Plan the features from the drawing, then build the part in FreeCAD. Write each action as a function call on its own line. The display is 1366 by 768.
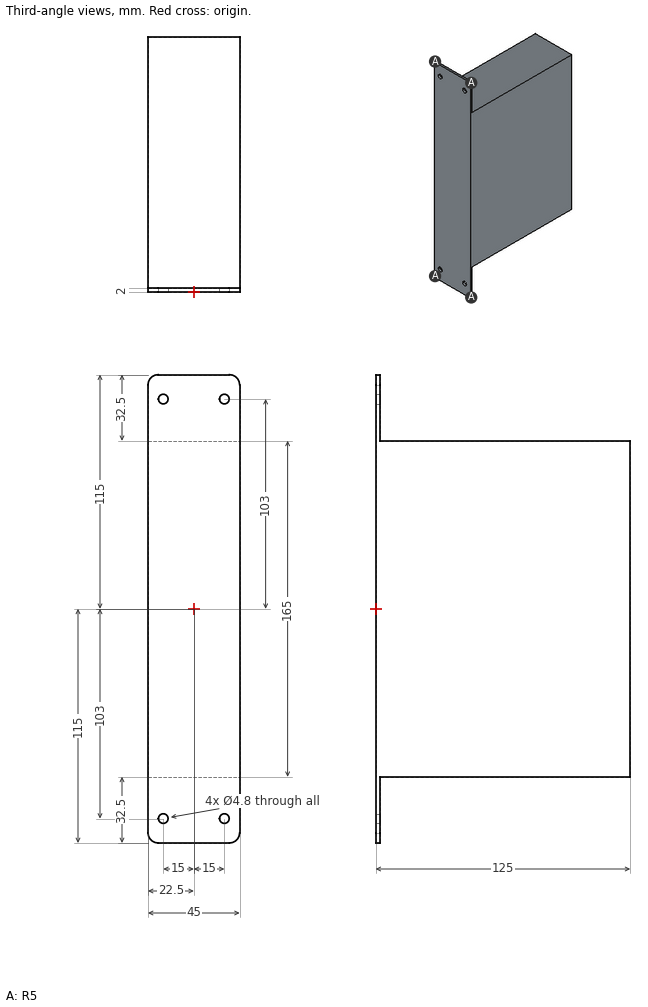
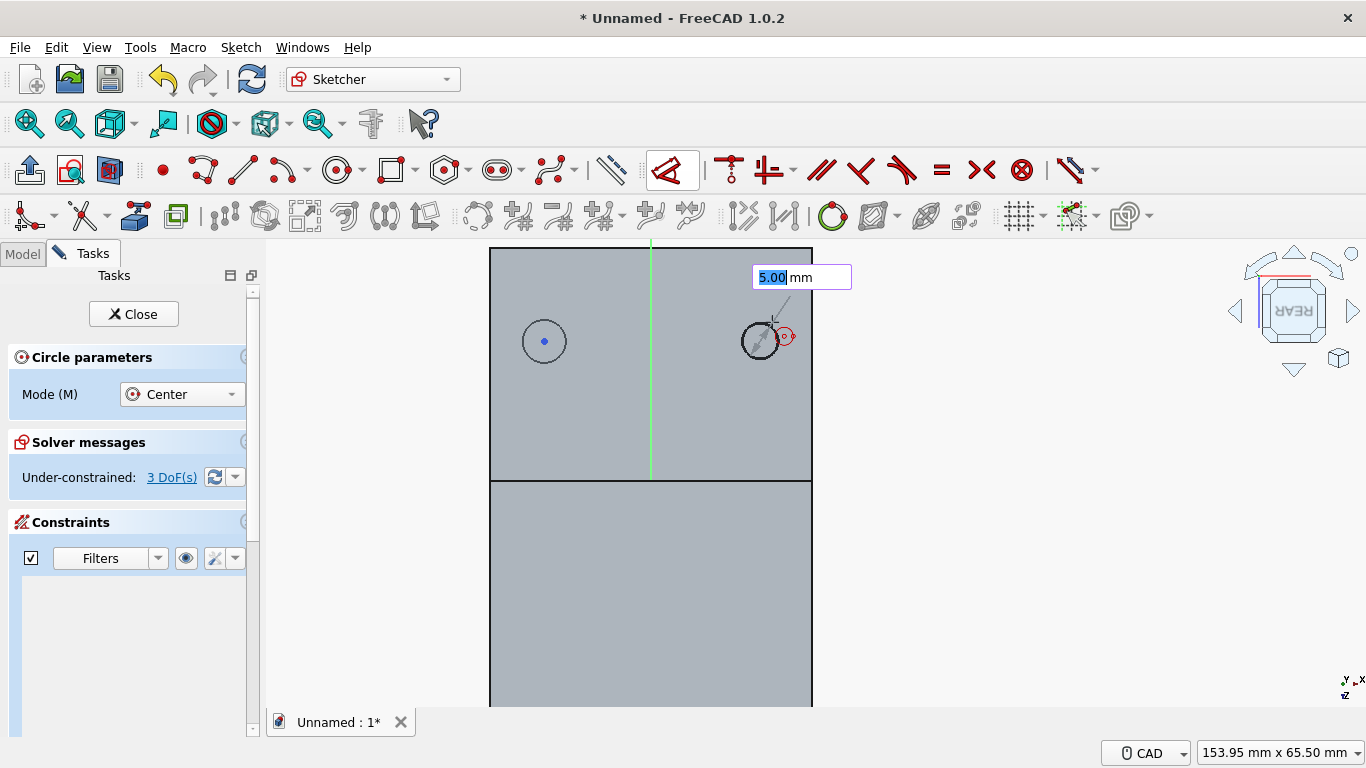
click(770, 322)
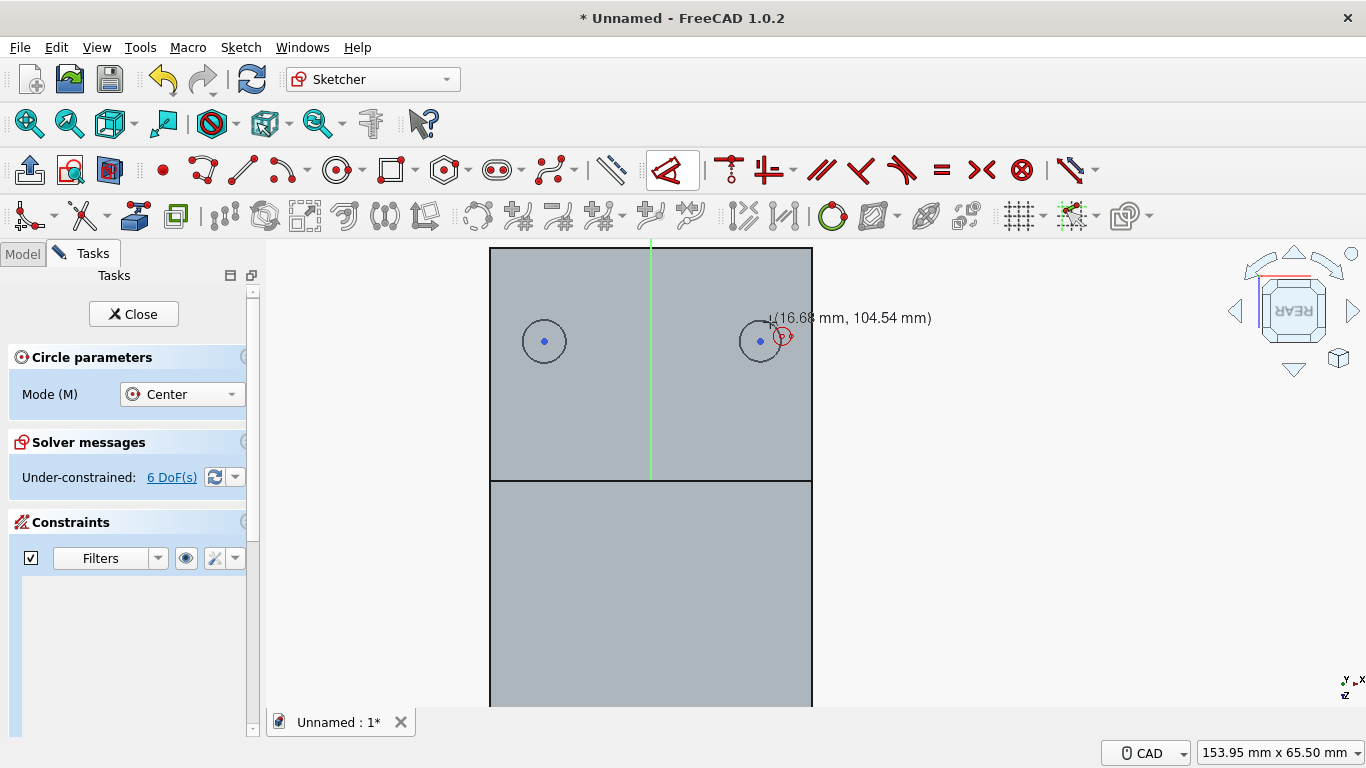
scroll(772, 322, down, 8)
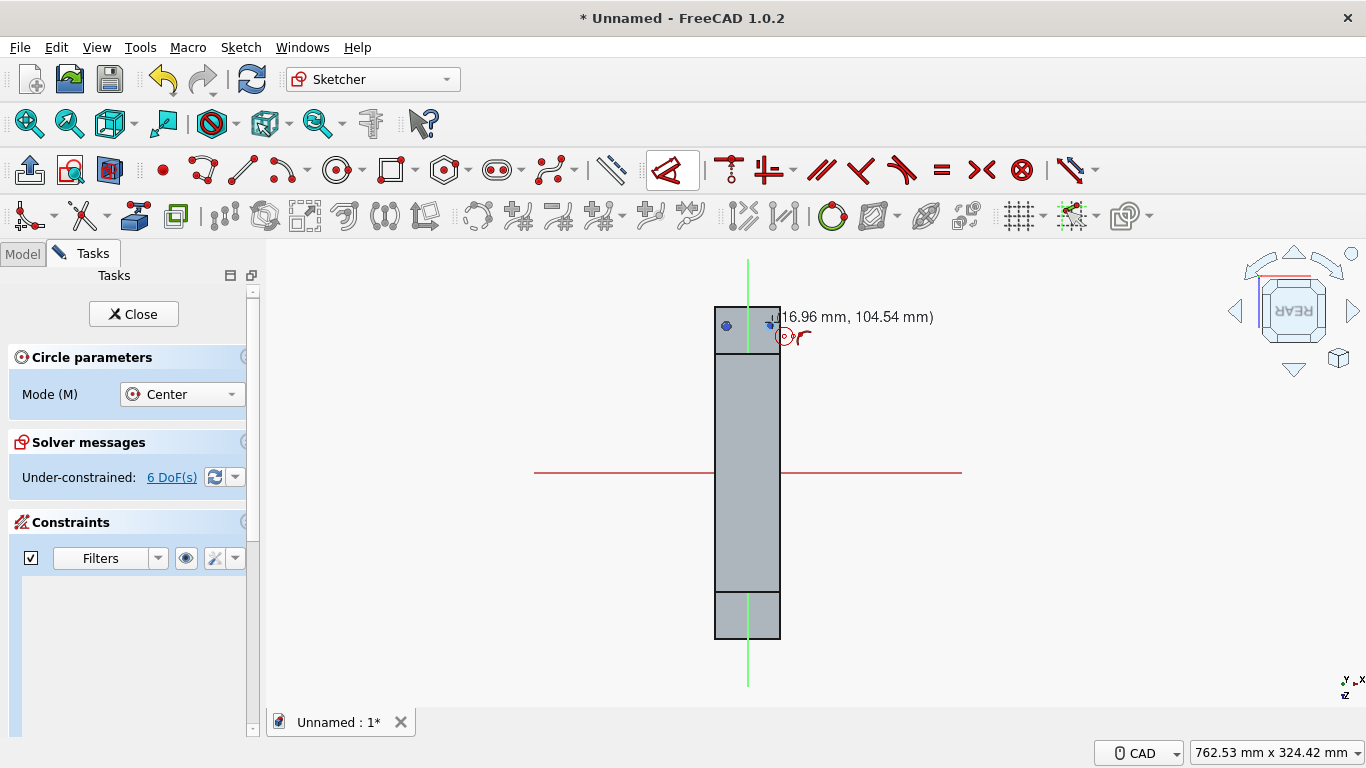
scroll(770, 622, up, 10)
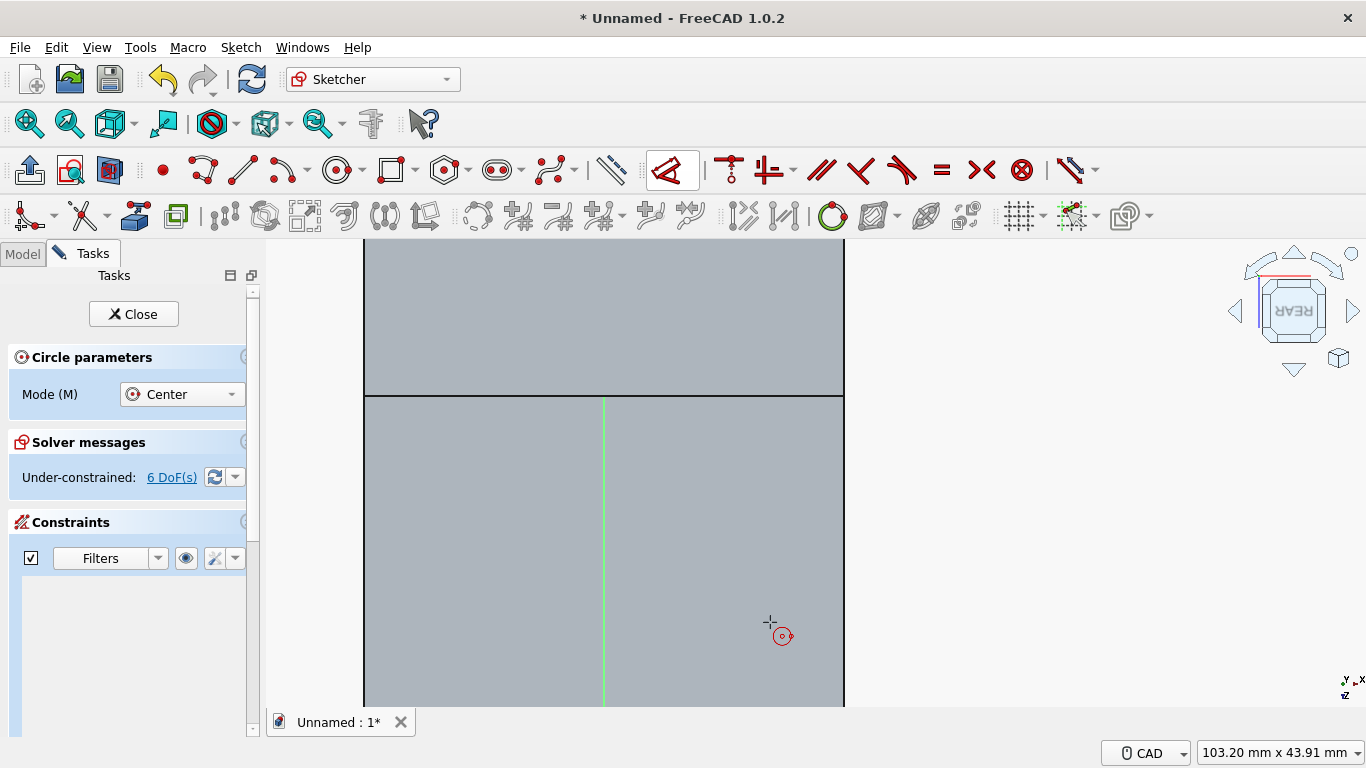
scroll(770, 623, down, 10)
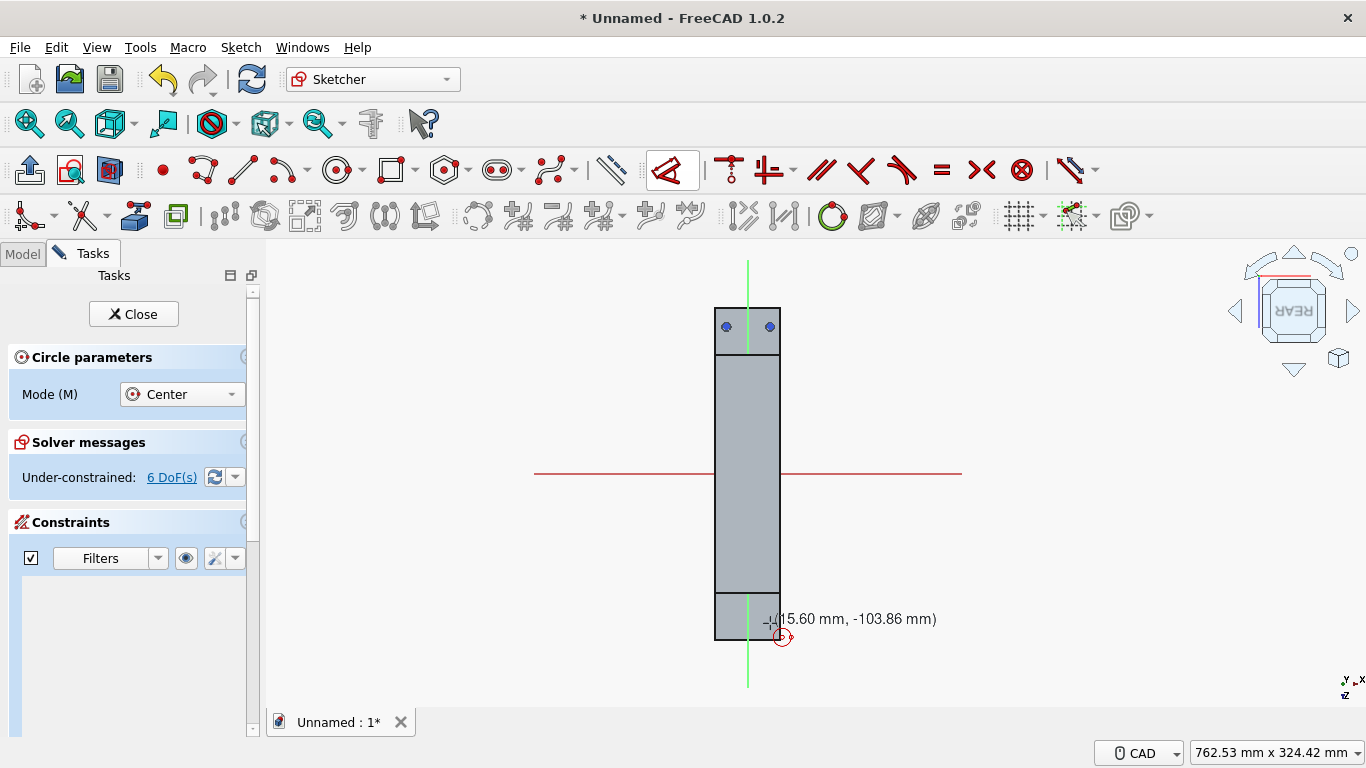
click(770, 623)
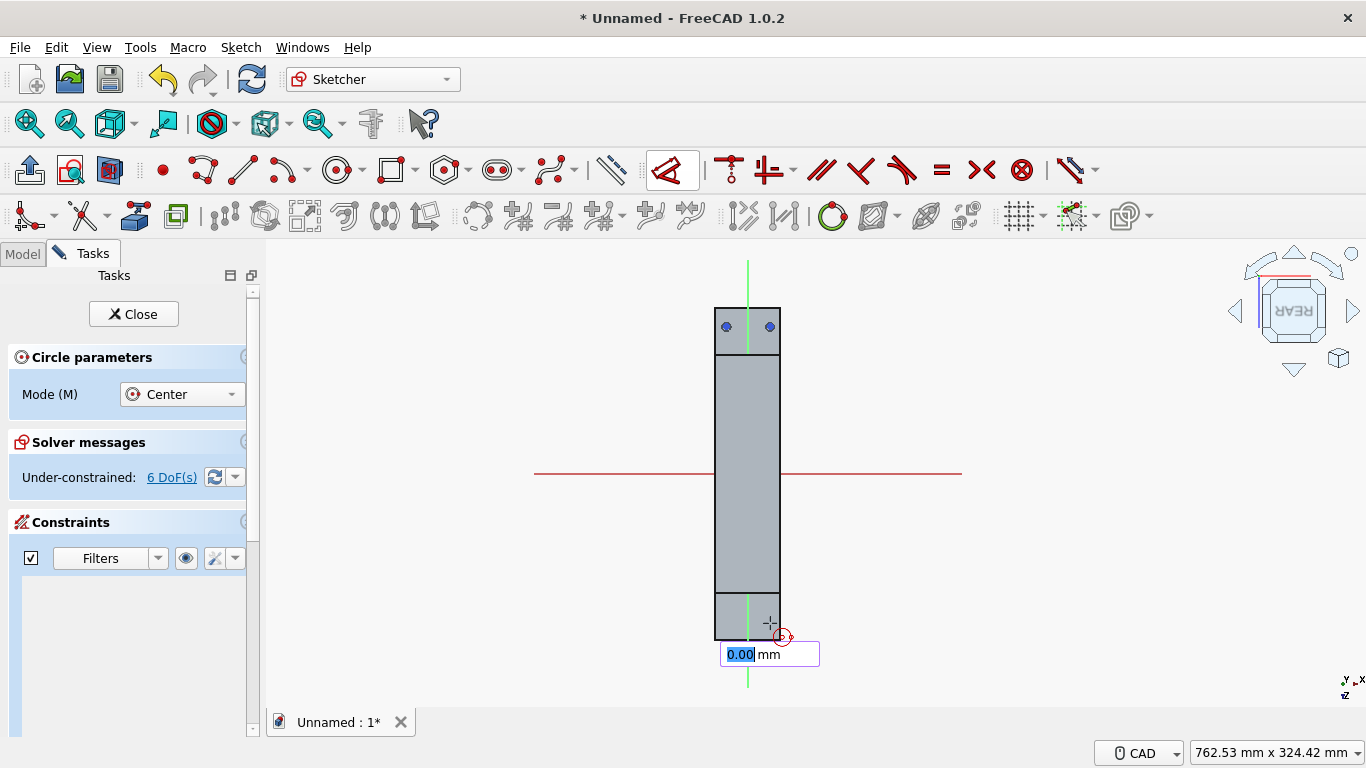
scroll(772, 620, up, 8)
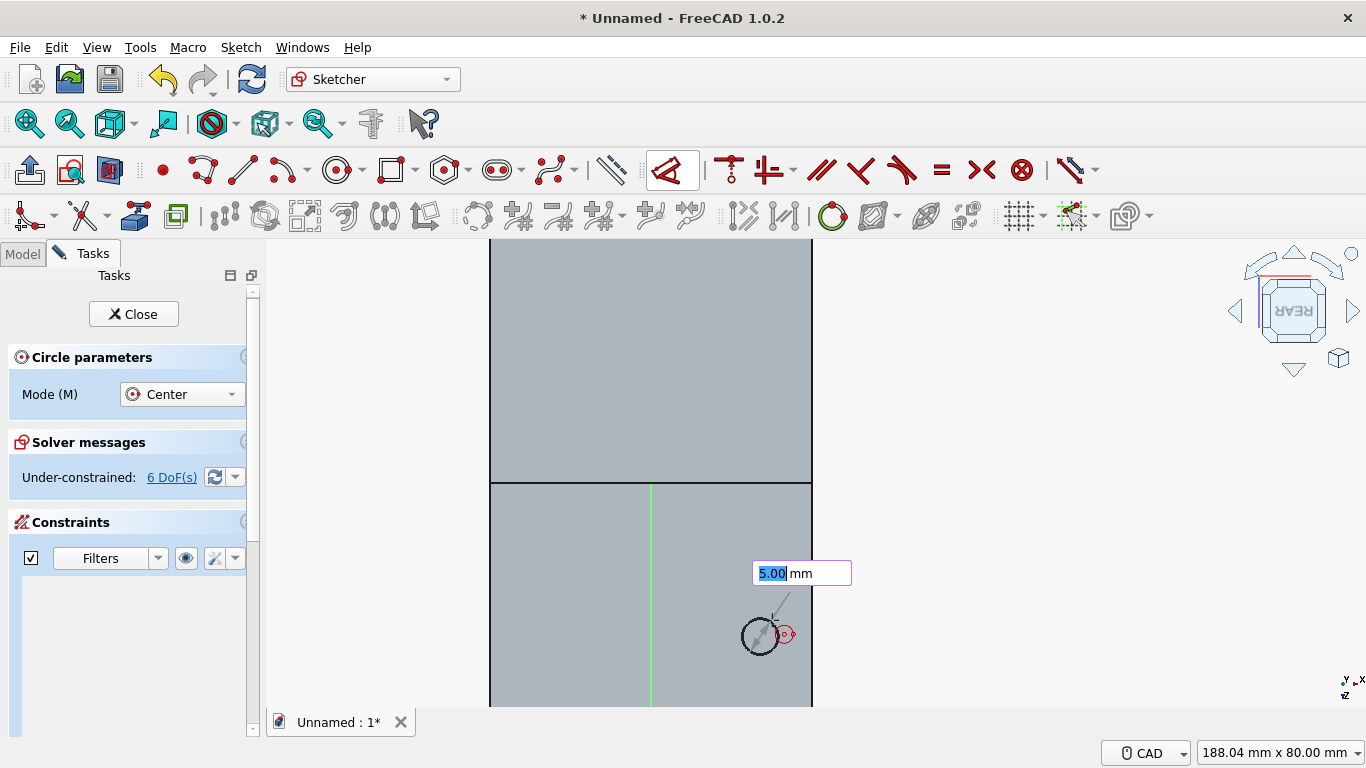
click(770, 618)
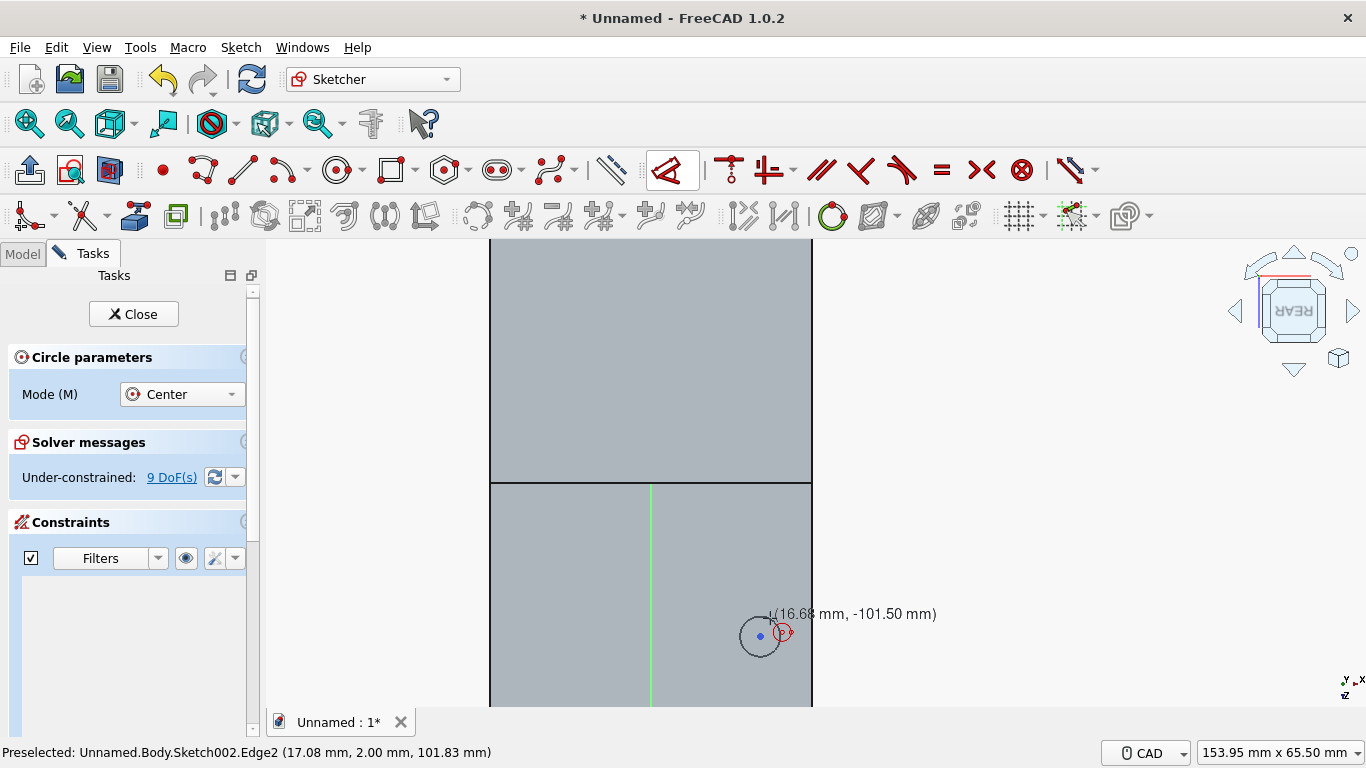
scroll(544, 630, up, 2)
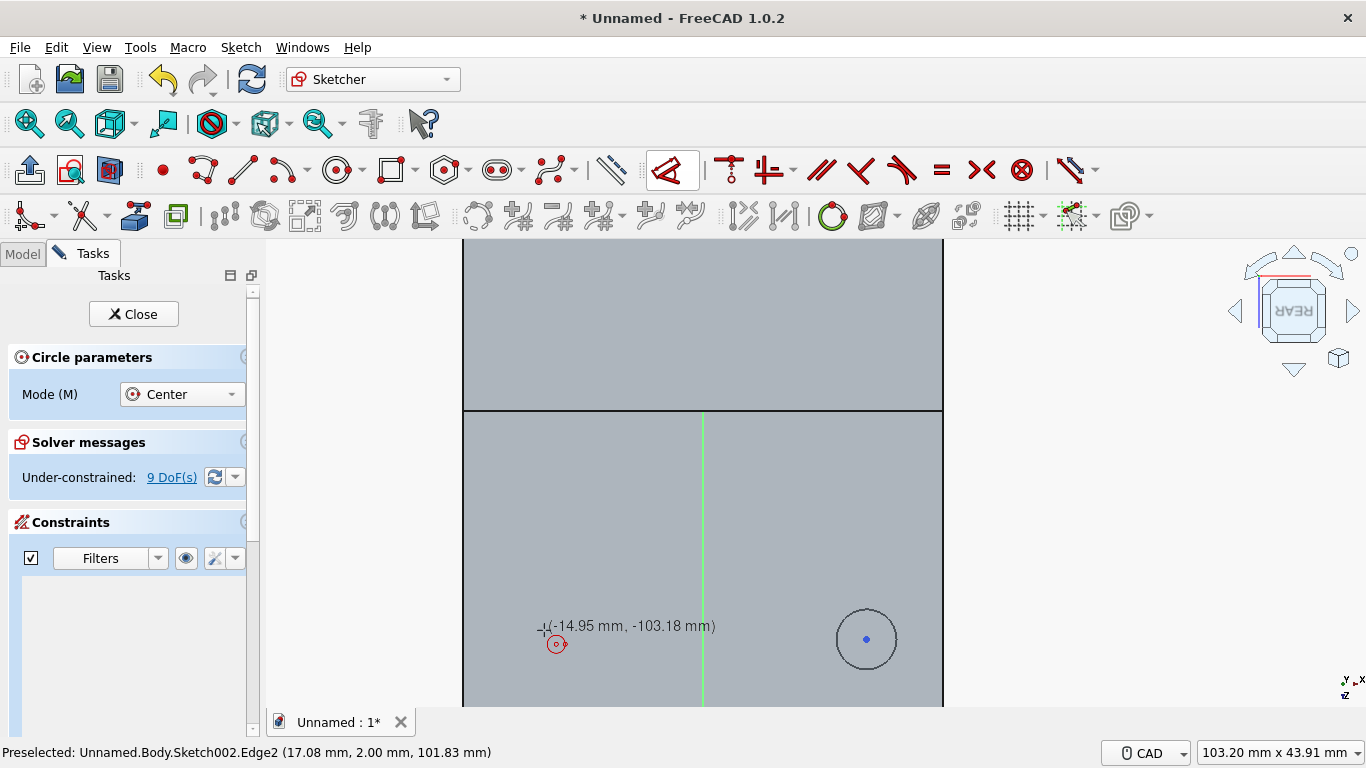
scroll(754, 620, down, 10)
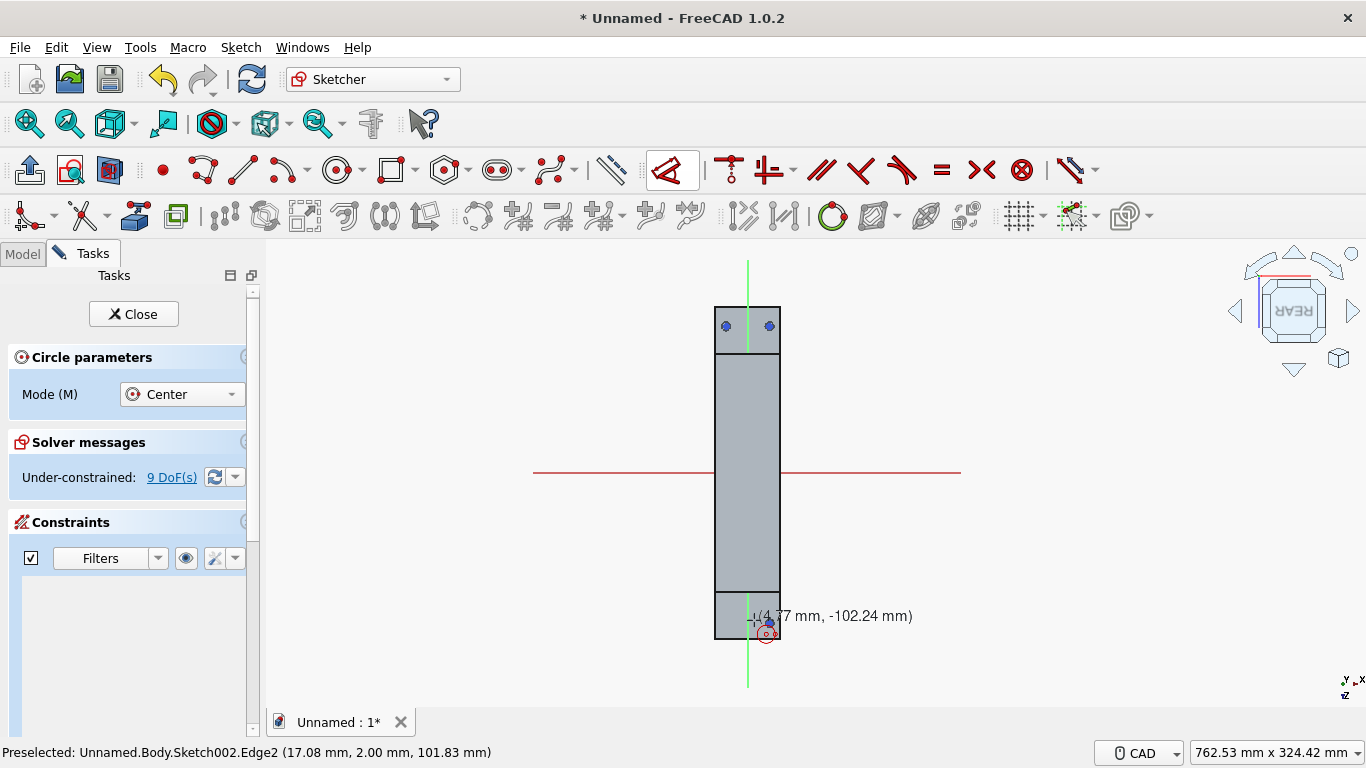
click(726, 622)